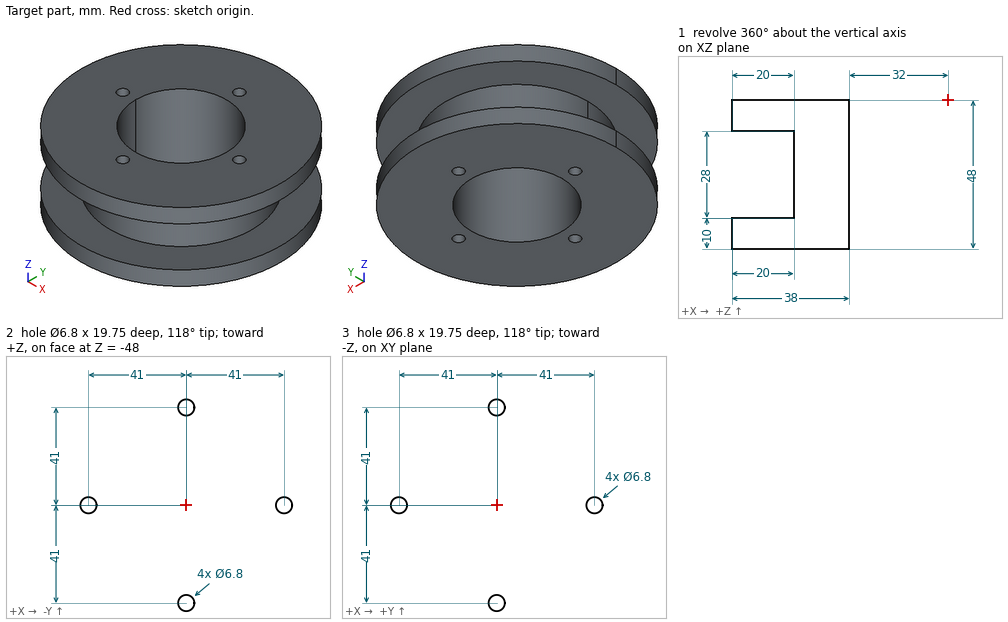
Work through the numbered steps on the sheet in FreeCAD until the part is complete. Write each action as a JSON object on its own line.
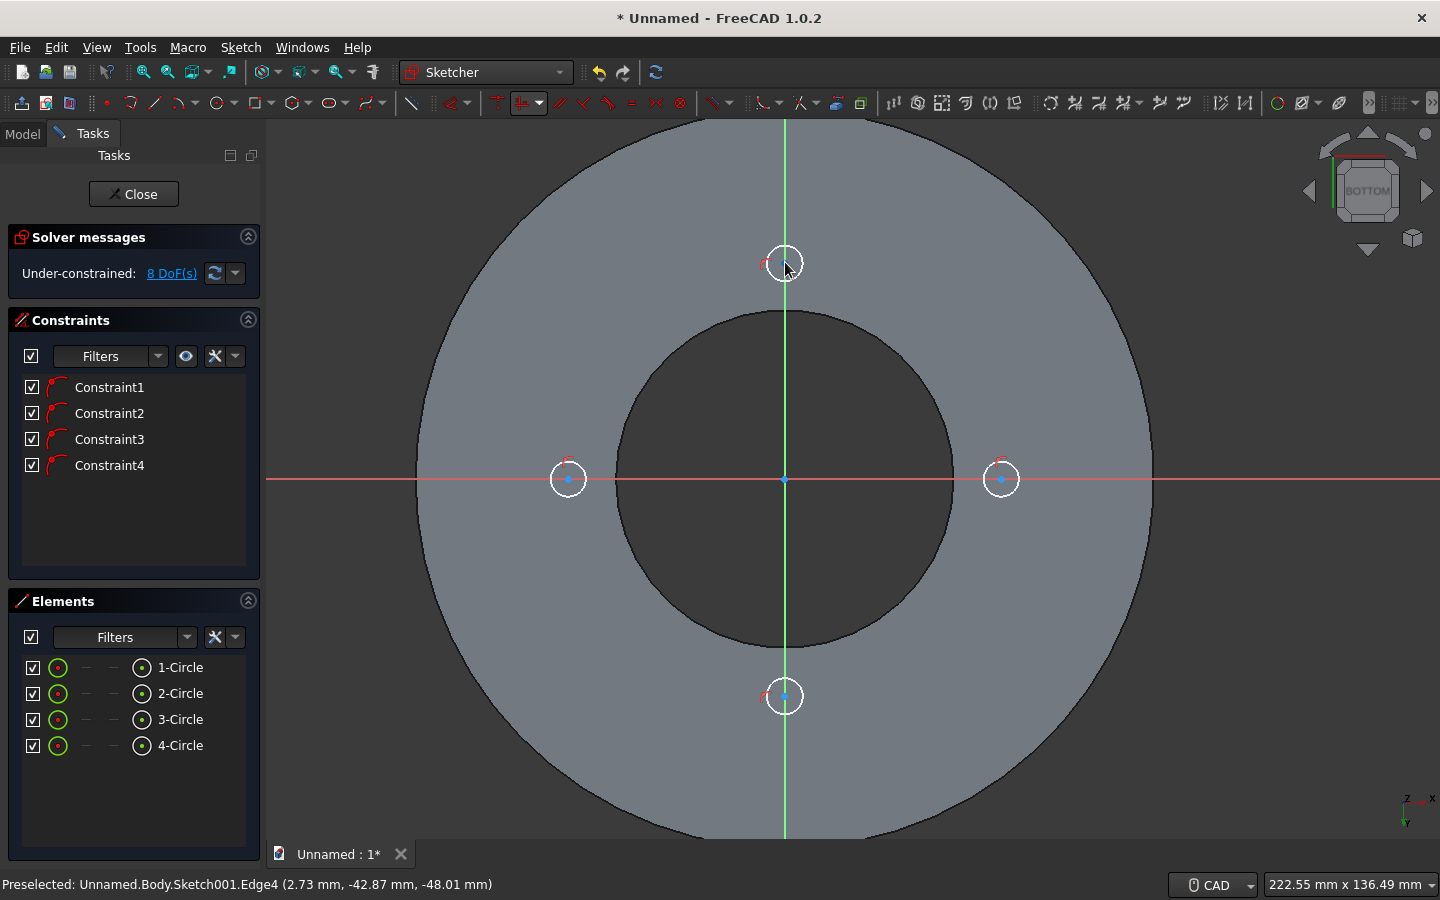
{"action": "left_click", "coordinate": [797, 683]}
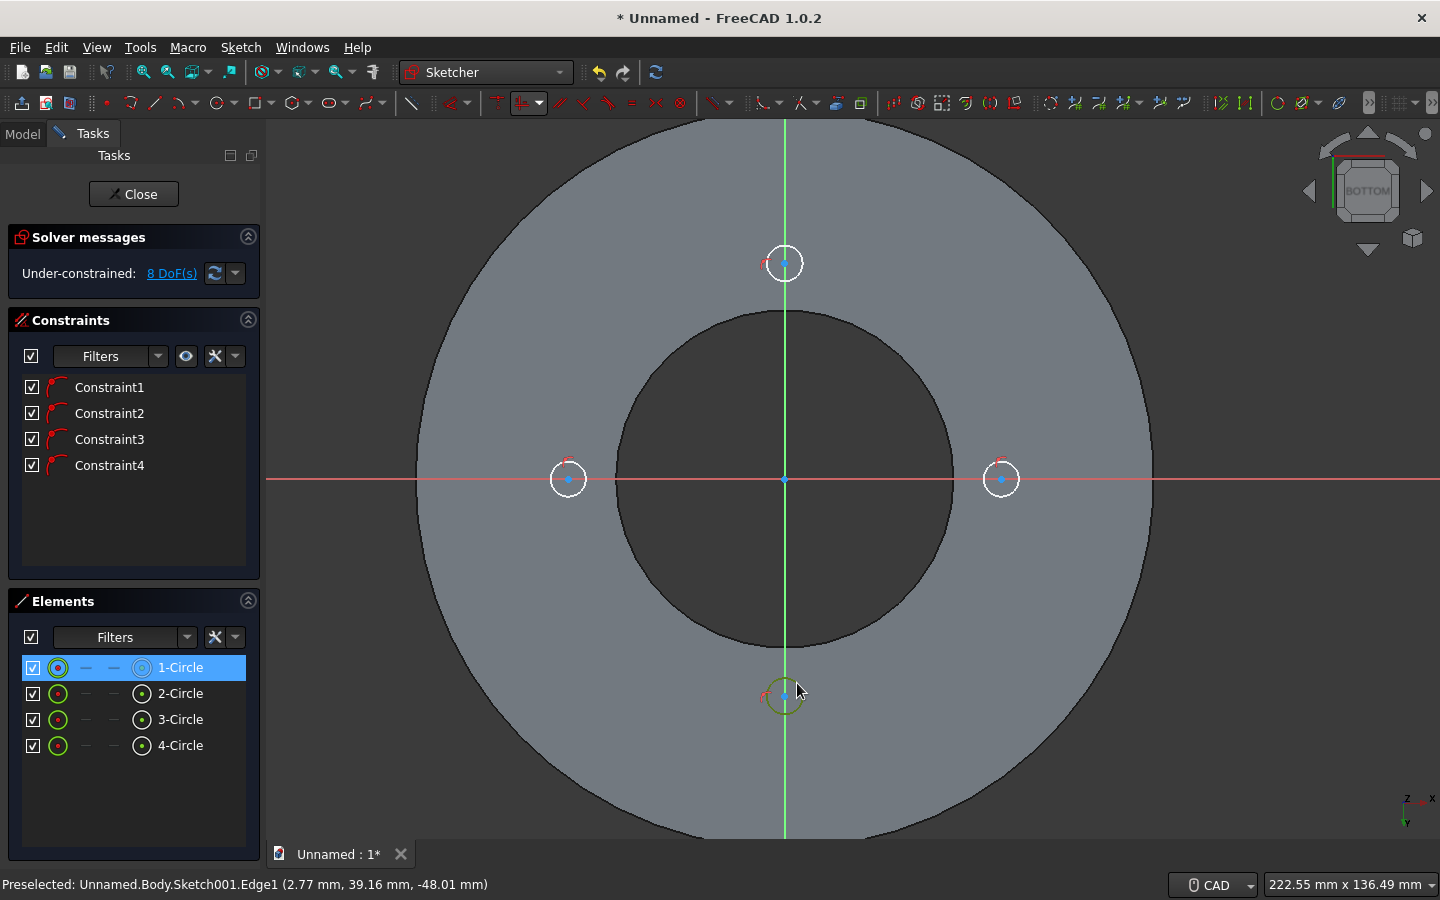
{"action": "left_click", "coordinate": [581, 467]}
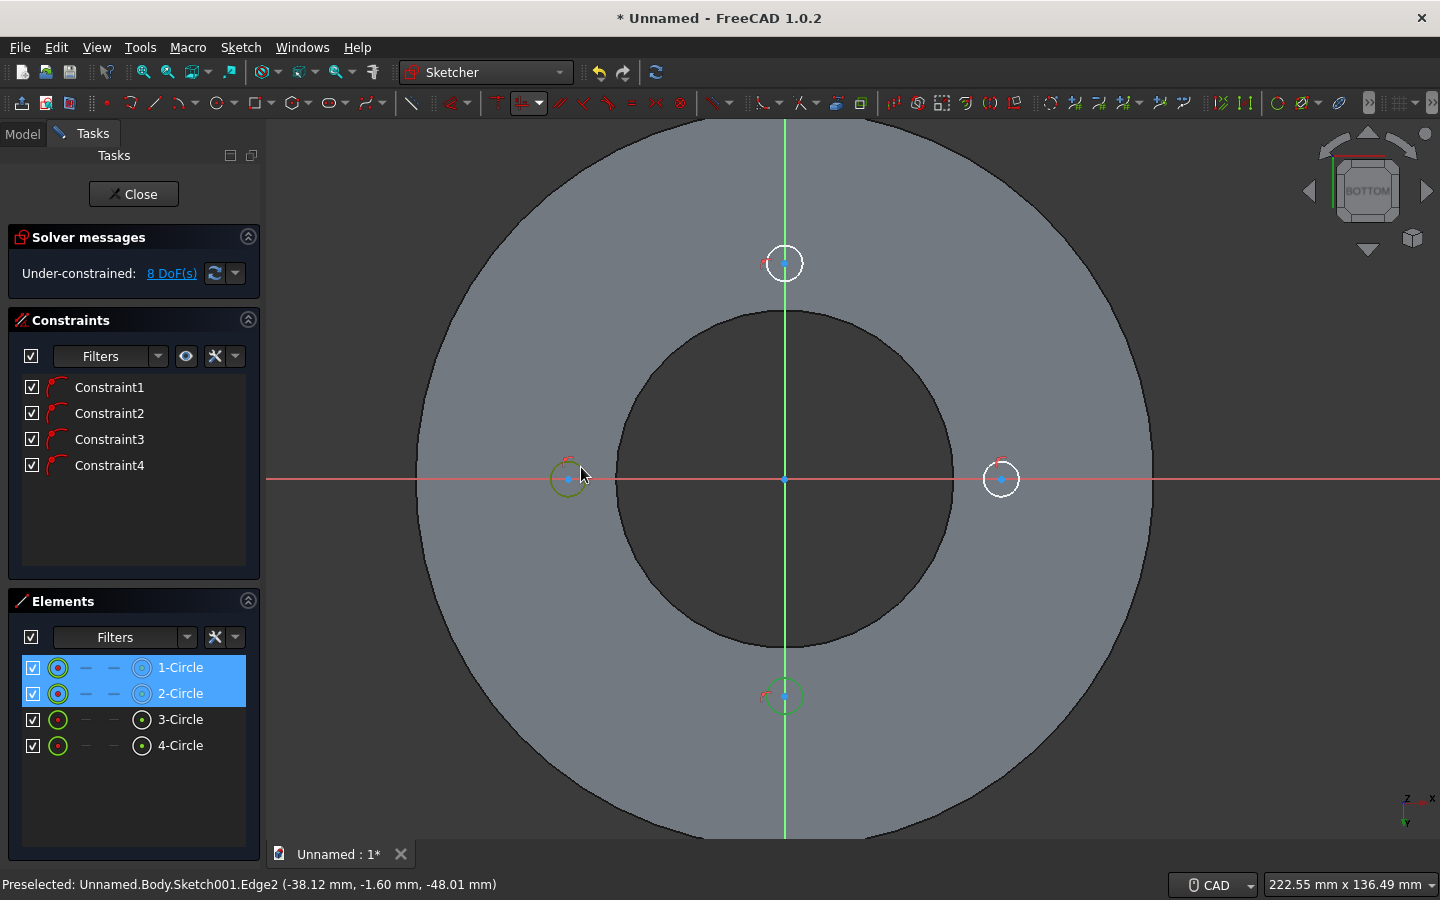
{"action": "left_click", "coordinate": [1014, 467]}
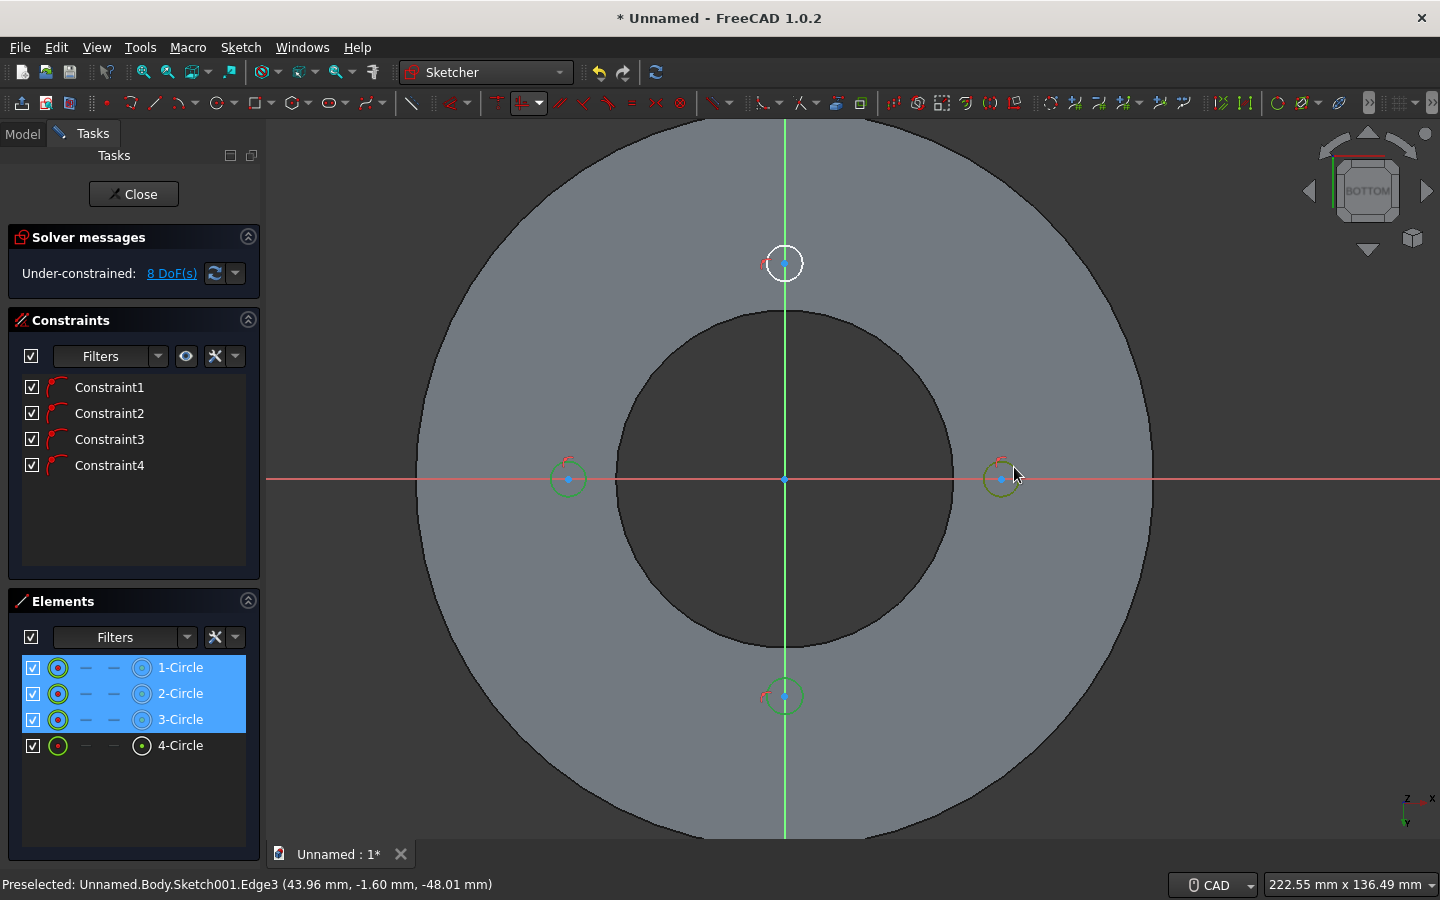
{"action": "left_click", "coordinate": [797, 251]}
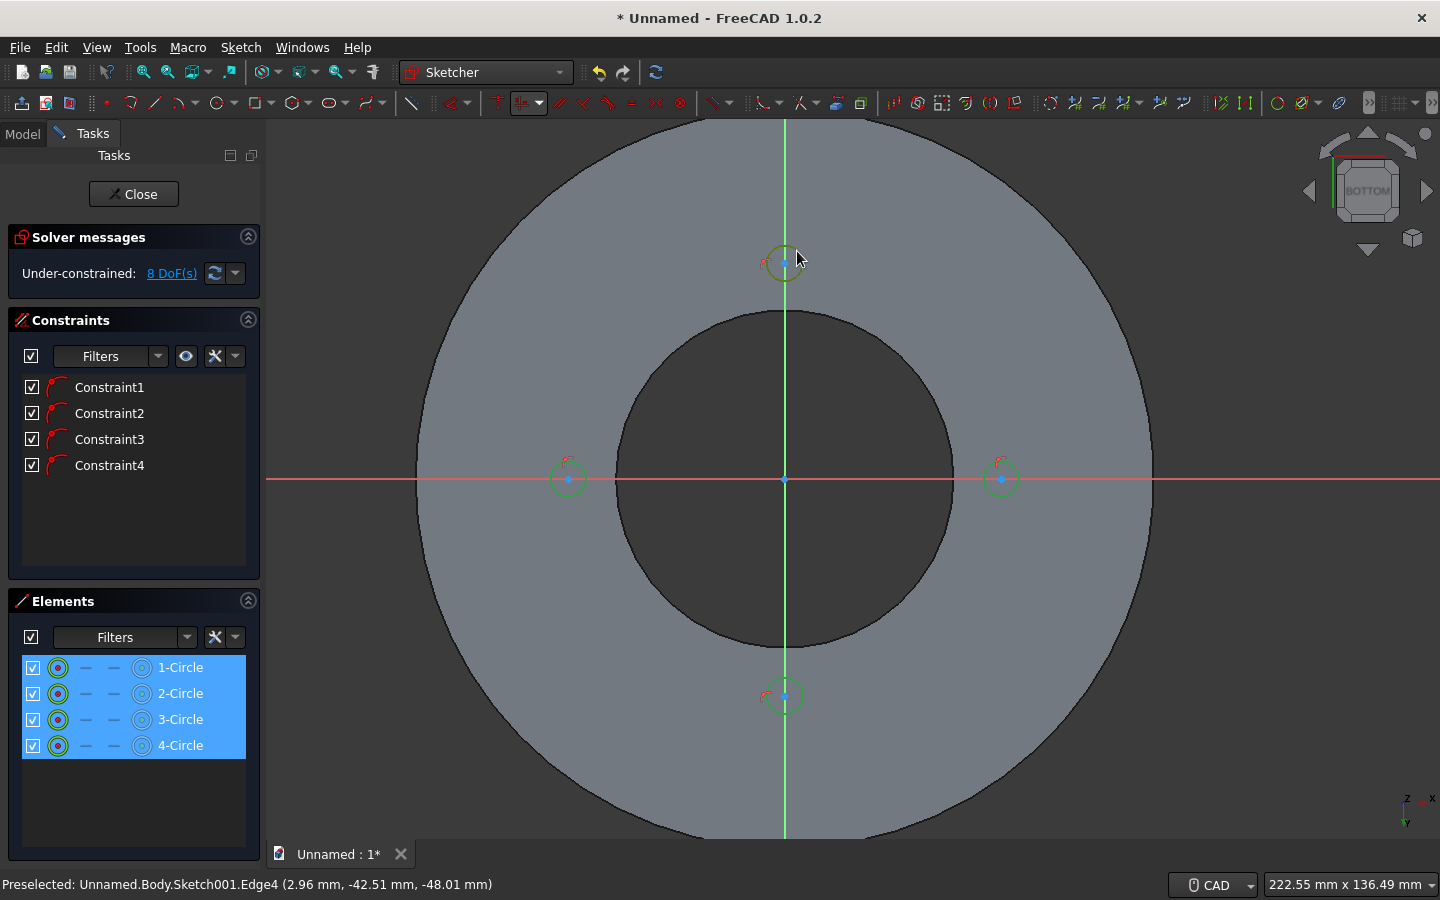
{"action": "left_click", "coordinate": [632, 104]}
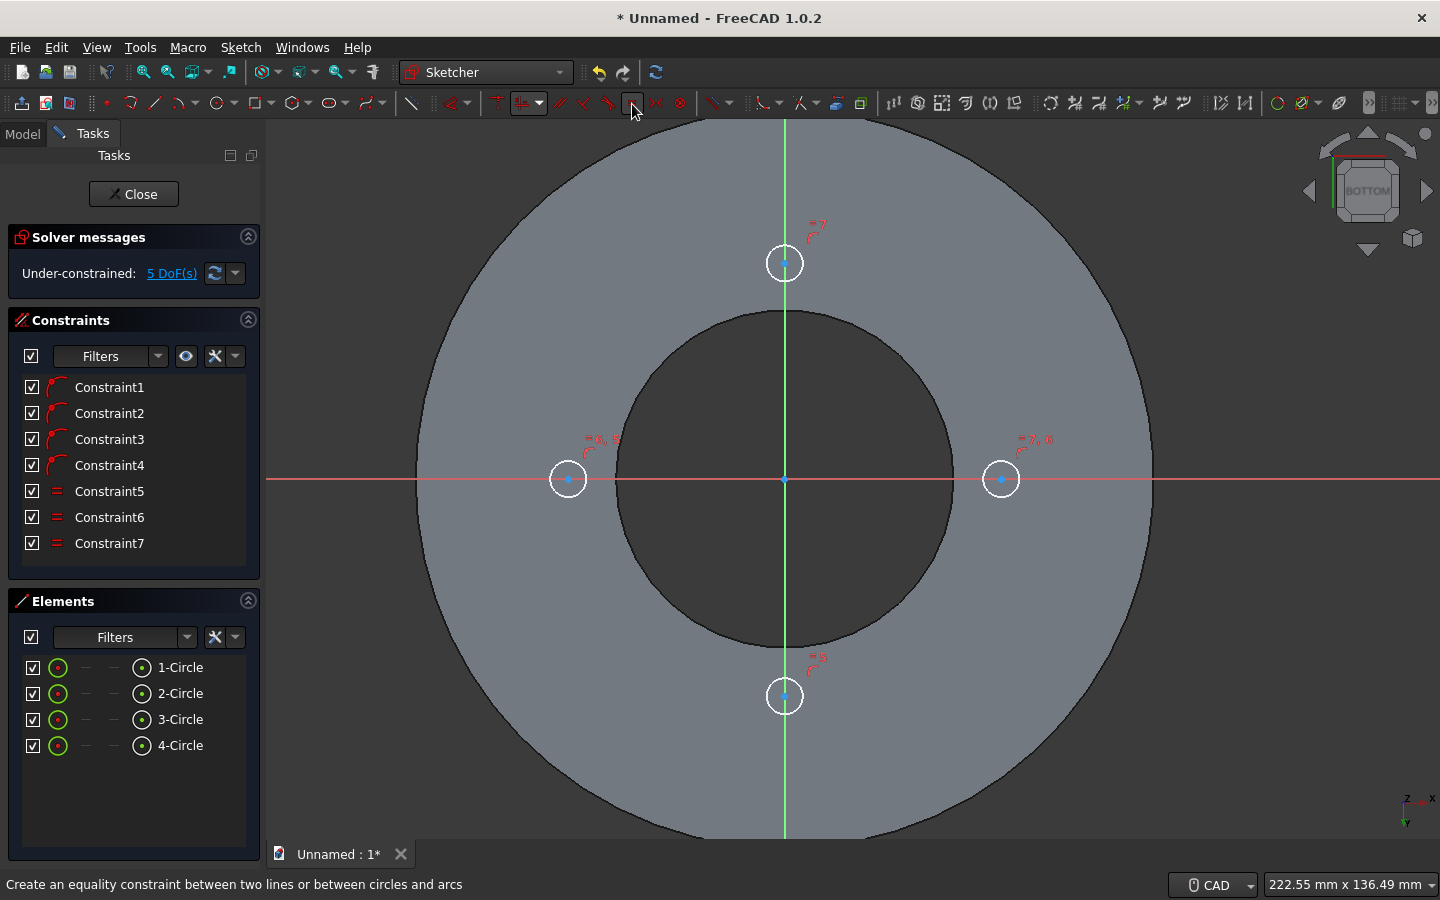
{"action": "left_click", "coordinate": [450, 104]}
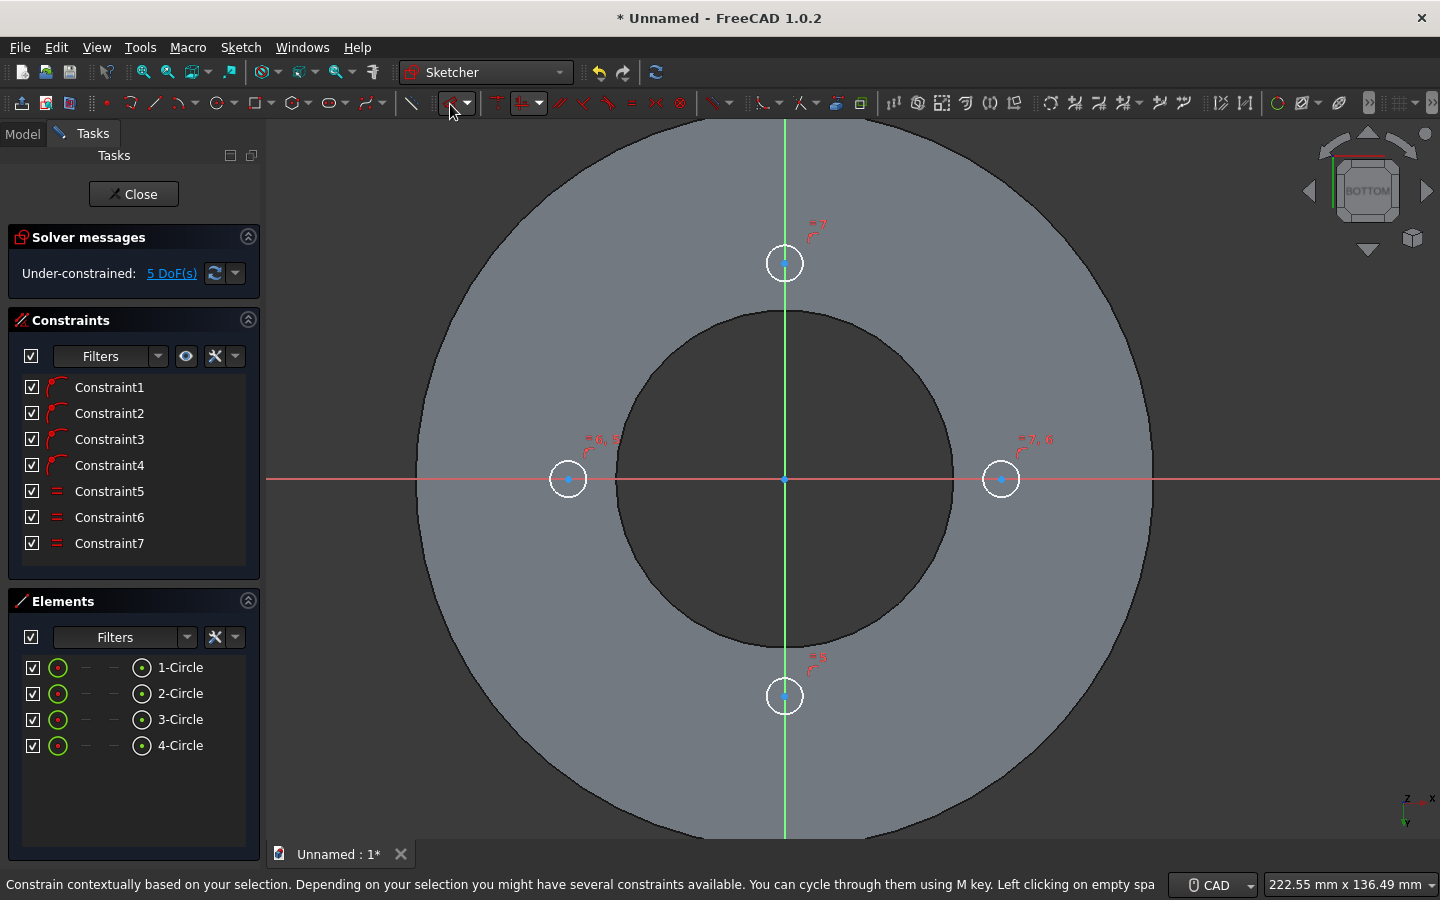
{"action": "left_click", "coordinate": [797, 683]}
{"action": "left_click", "coordinate": [819, 659]}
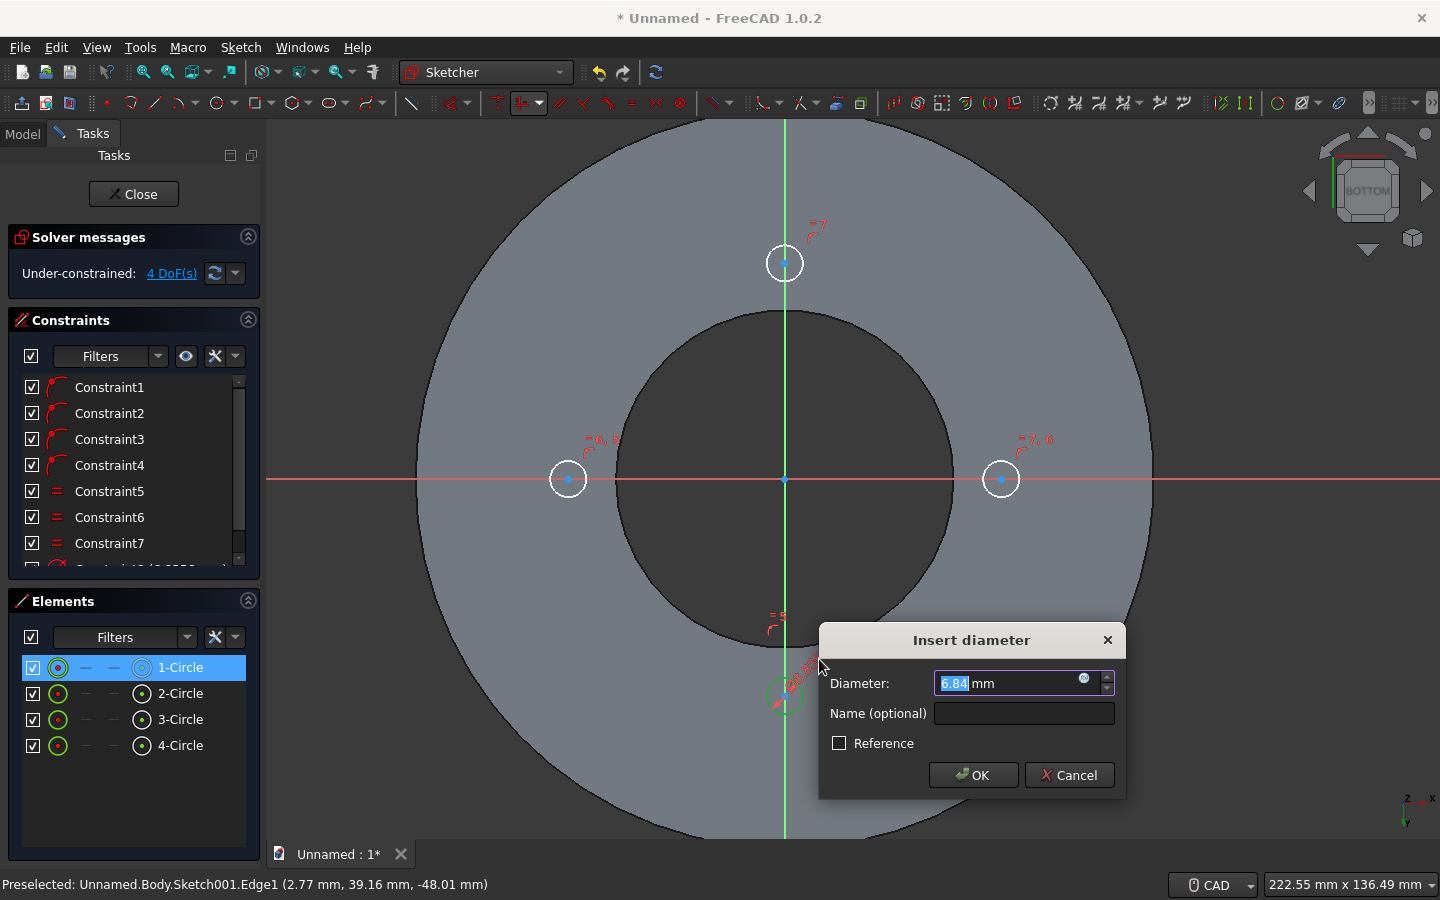
{"action": "type", "text": "6.8"}
{"action": "key", "text": "Return"}